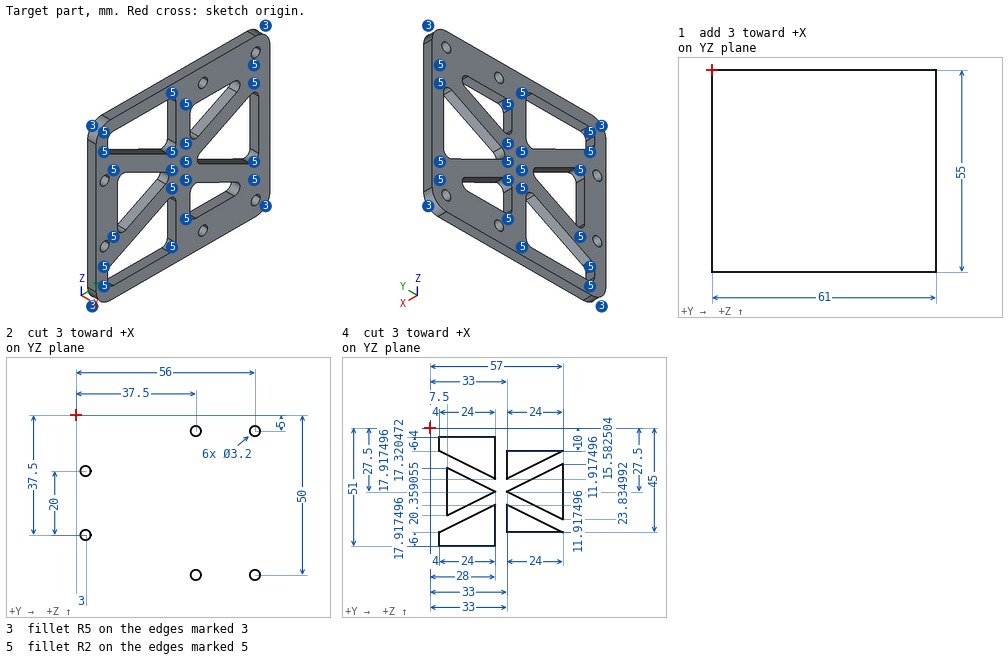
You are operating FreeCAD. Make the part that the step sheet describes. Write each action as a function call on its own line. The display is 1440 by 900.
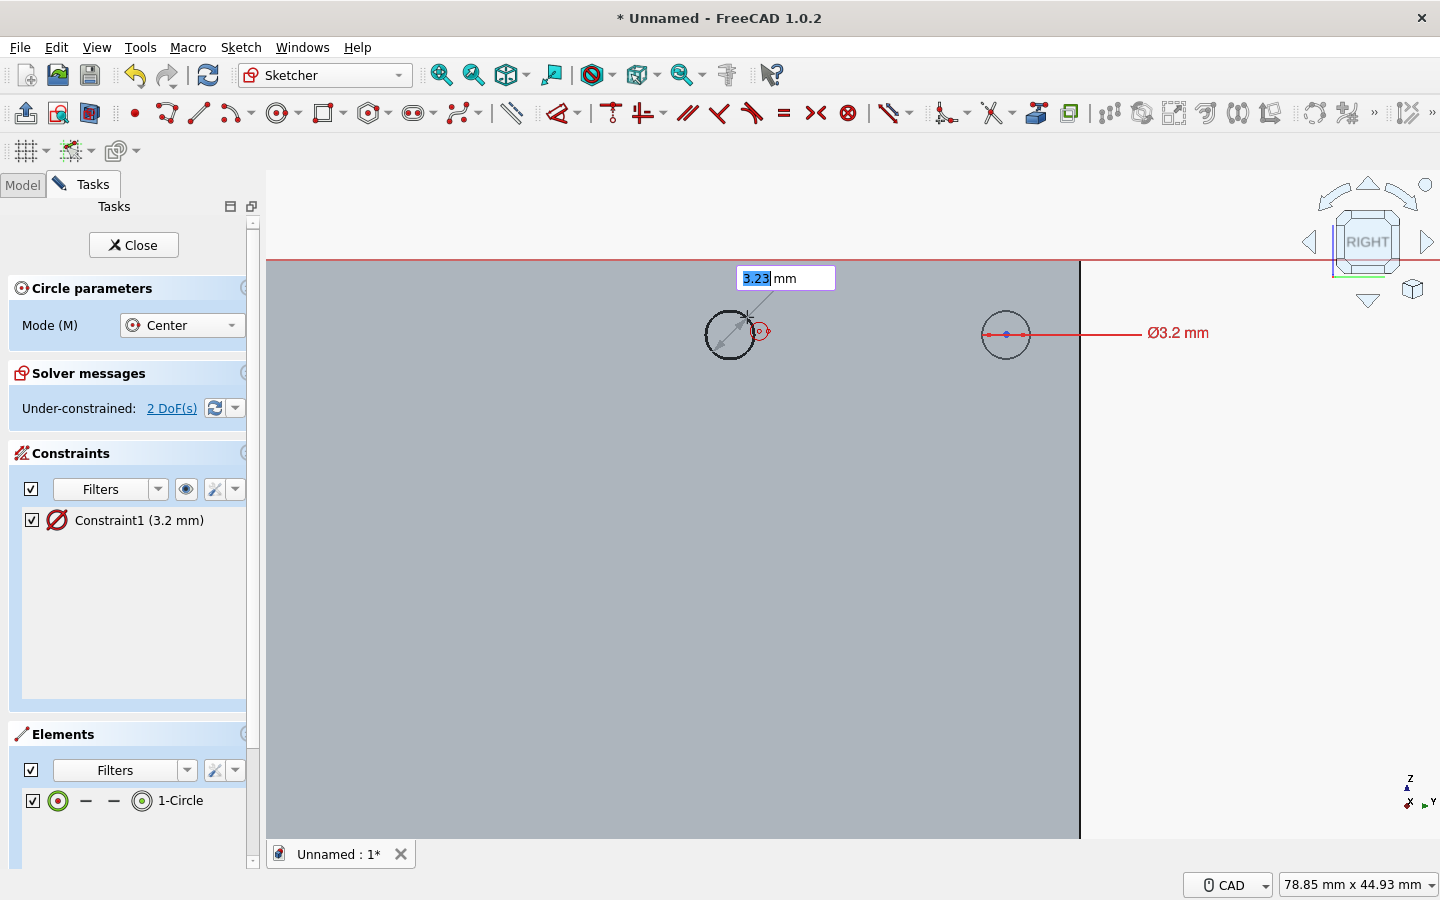
text(3.2)
key(Return)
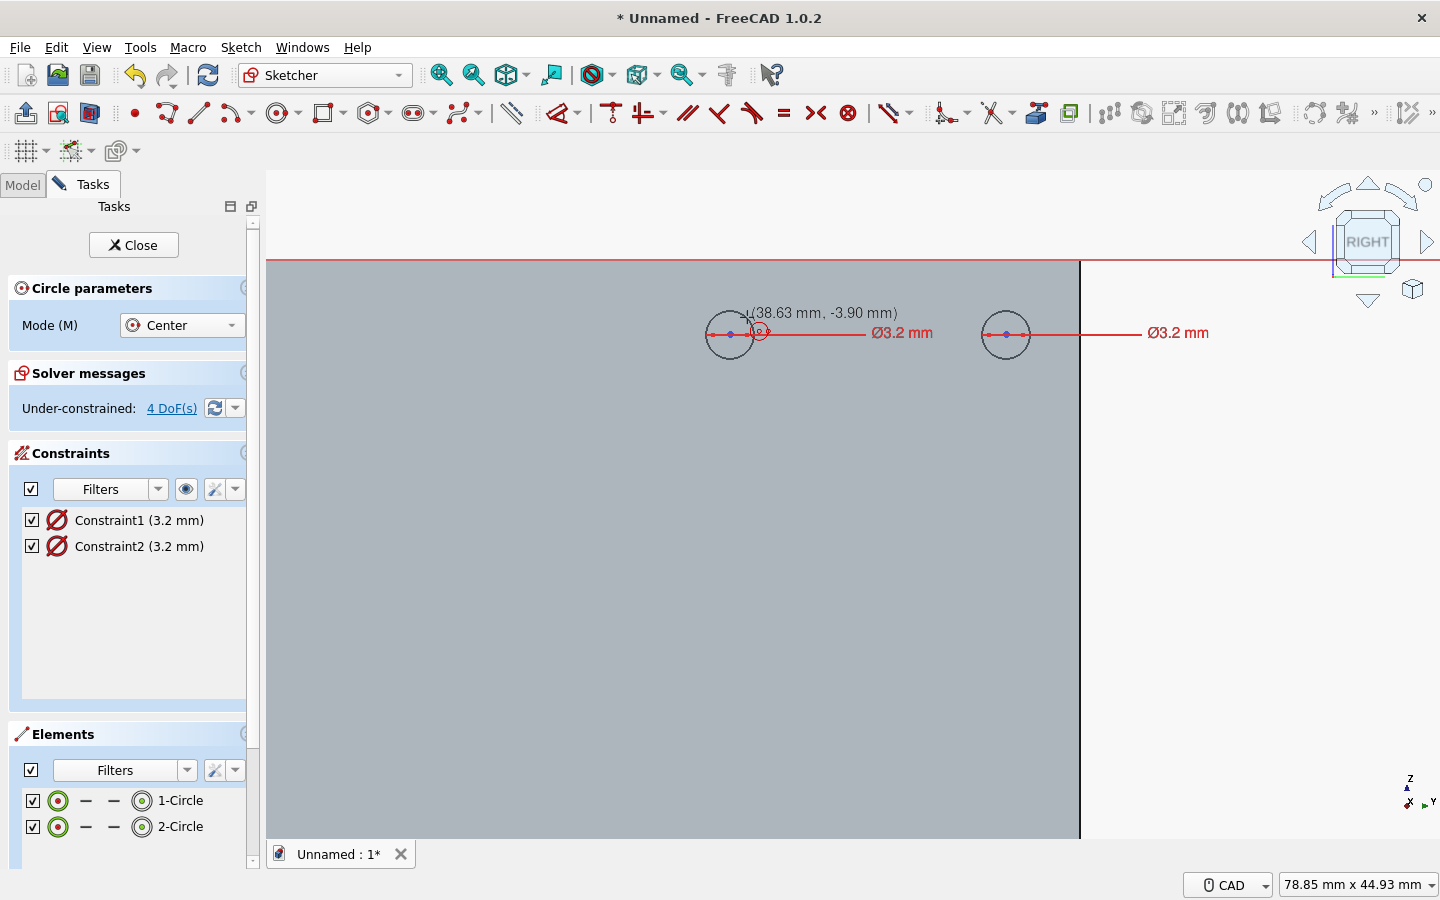
scroll(1008, 335, down, 3)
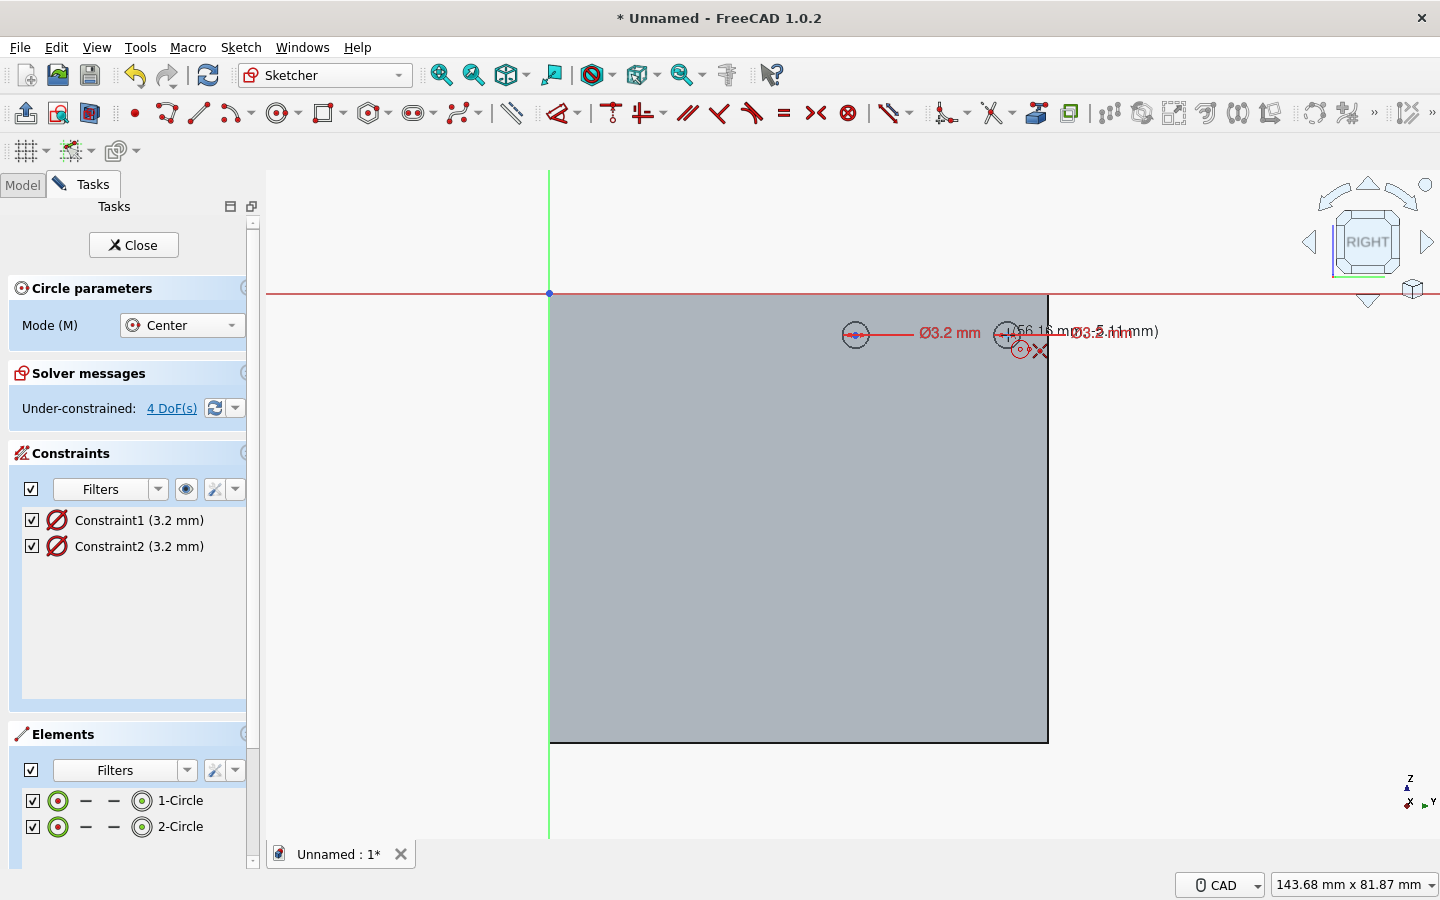
scroll(1007, 702, up, 3)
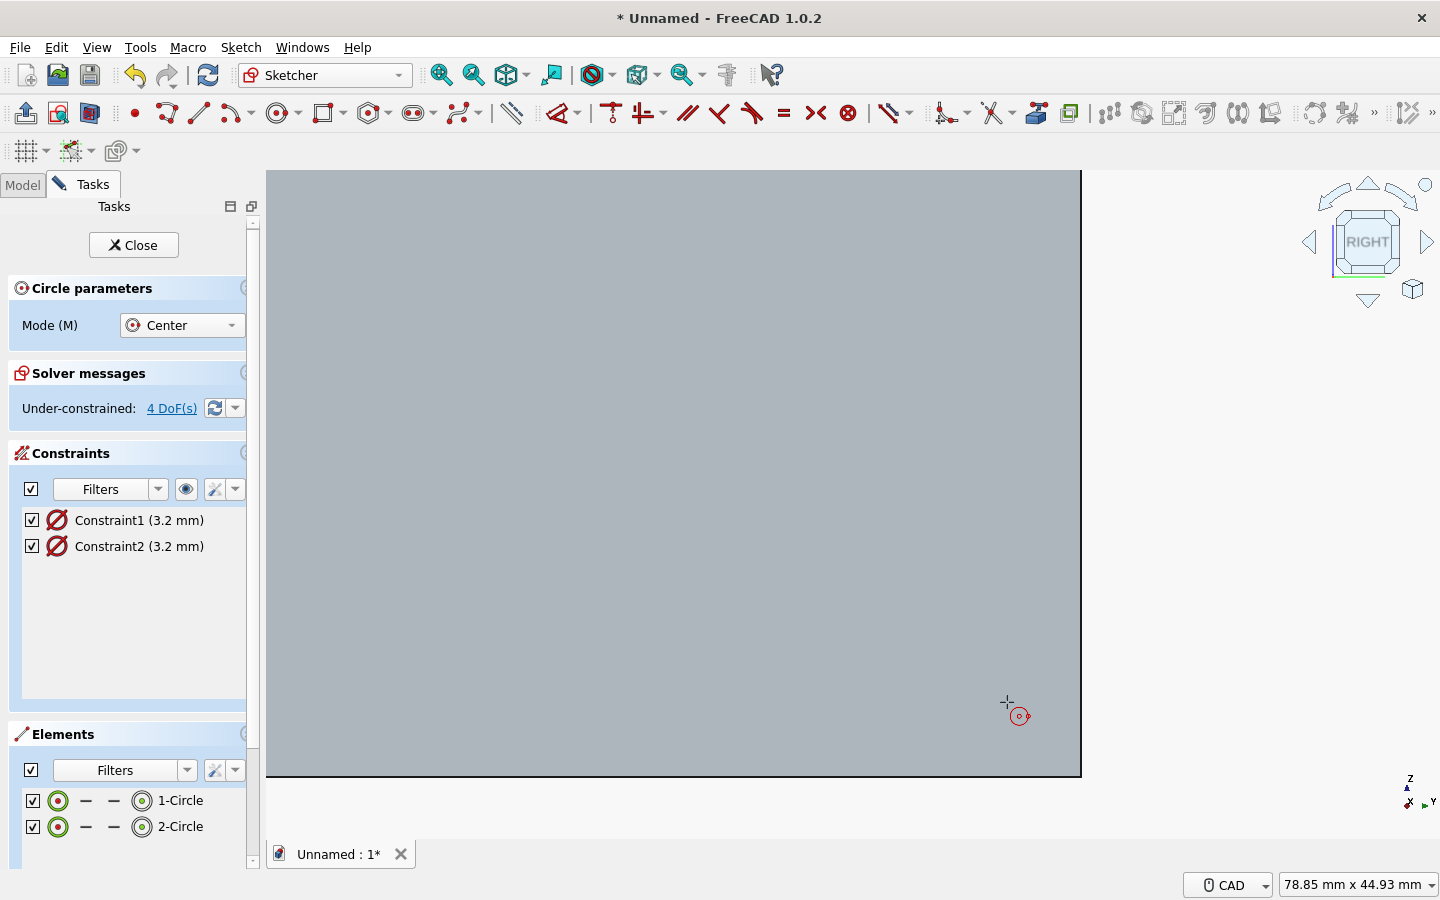
click(1006, 702)
move(1023, 685)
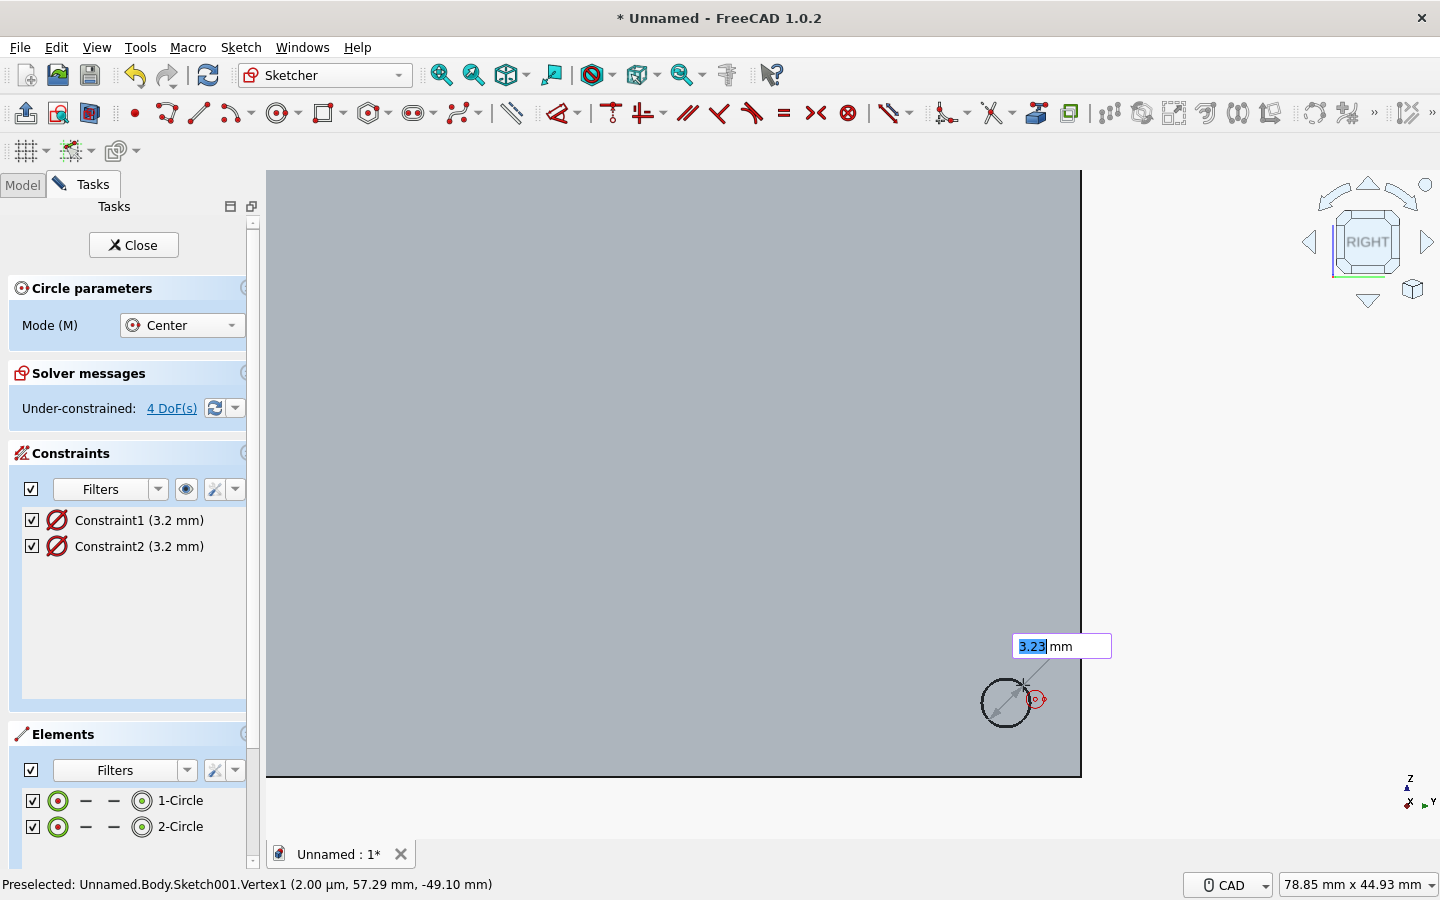
text(3.2)
key(Return)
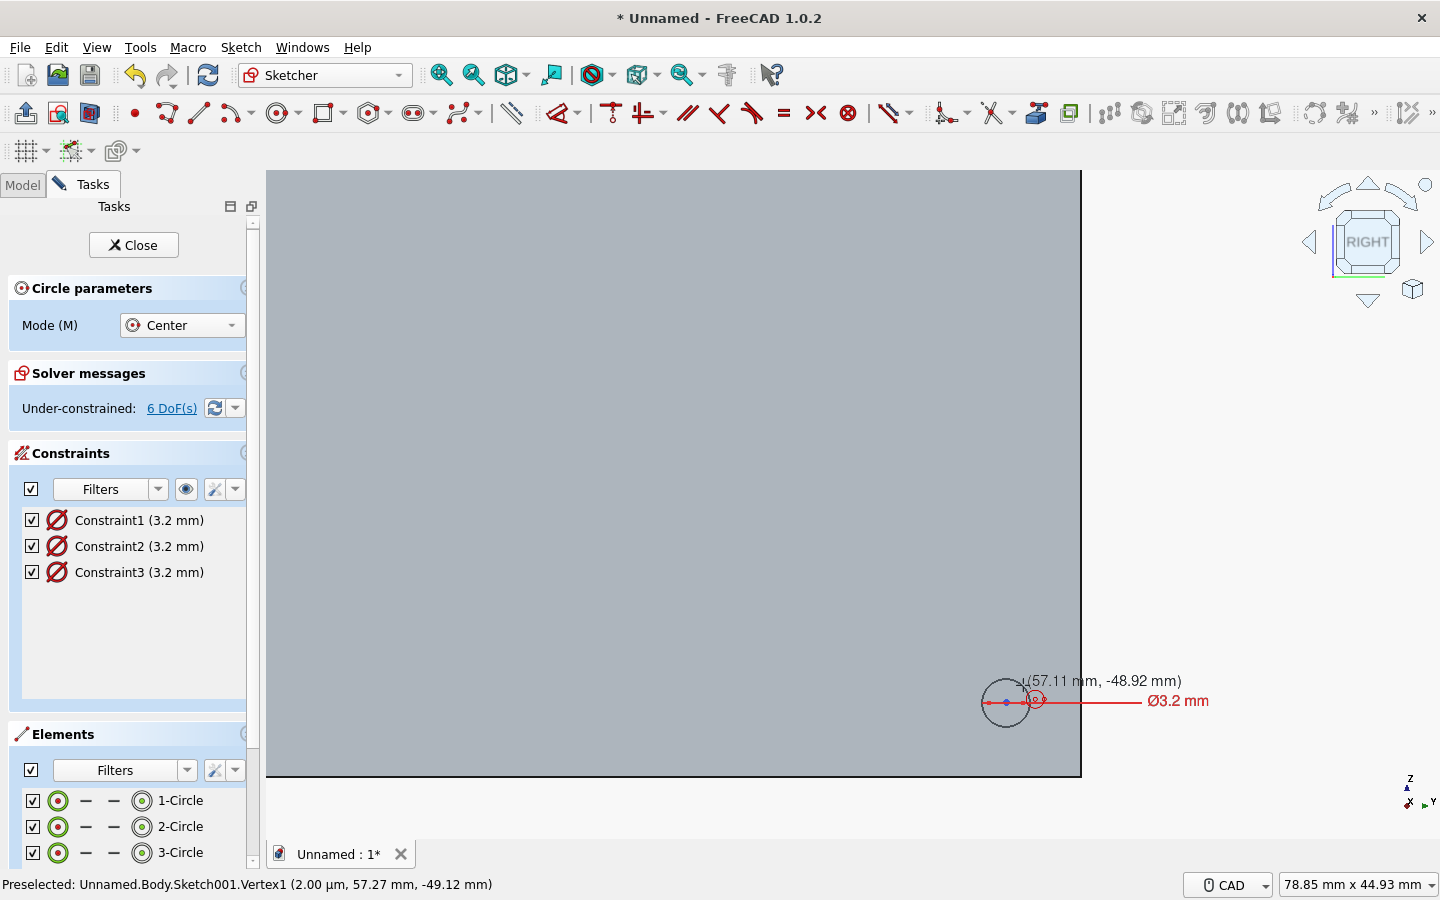
click(731, 702)
move(748, 685)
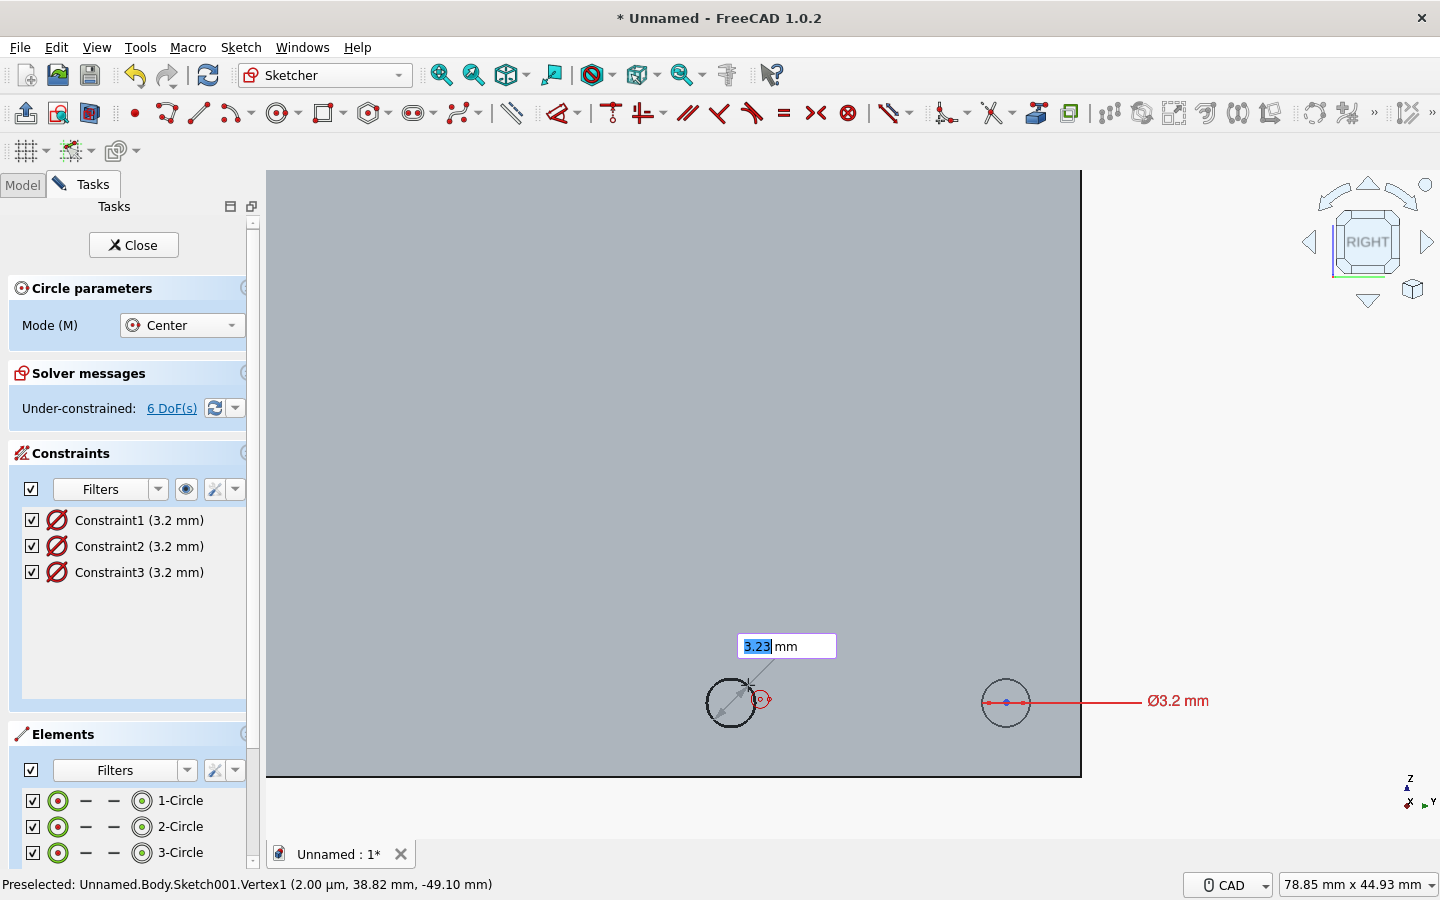
text(3.2)
key(Return)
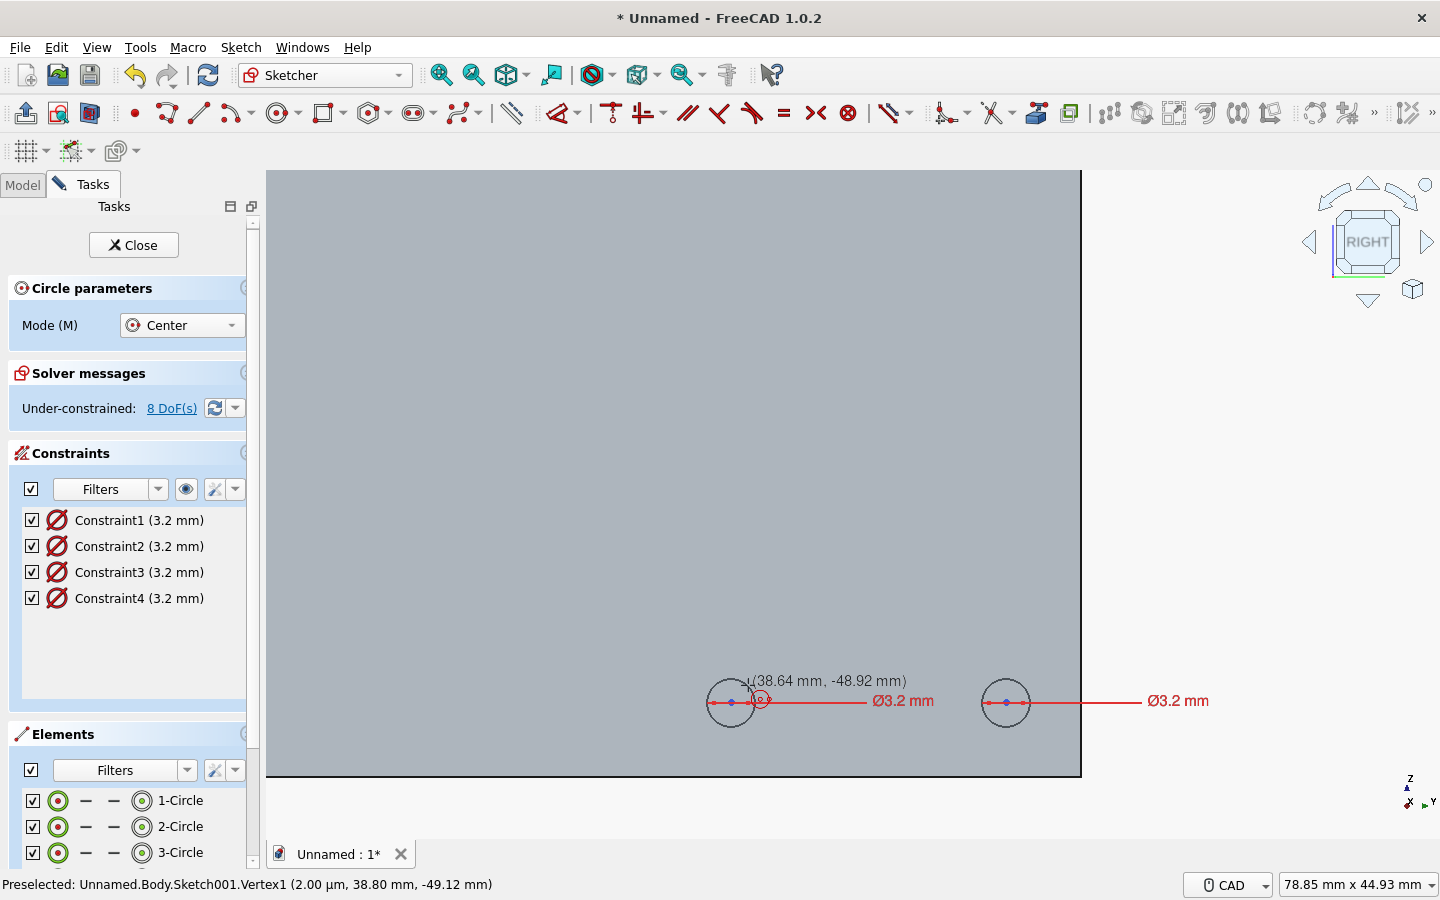
scroll(1007, 702, down, 3)